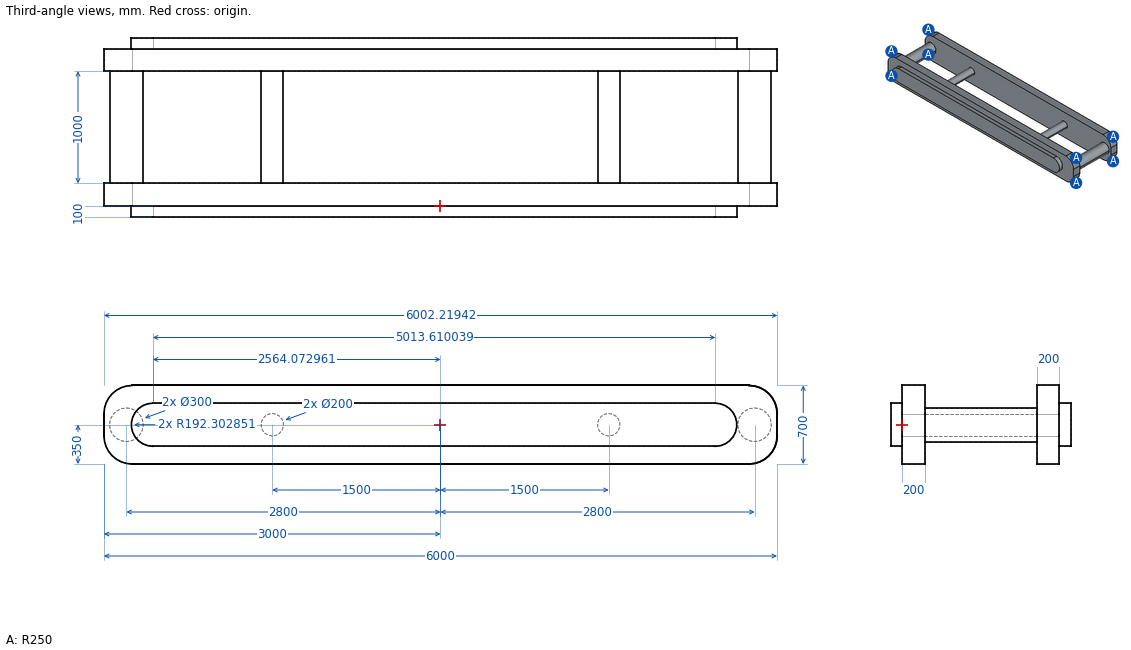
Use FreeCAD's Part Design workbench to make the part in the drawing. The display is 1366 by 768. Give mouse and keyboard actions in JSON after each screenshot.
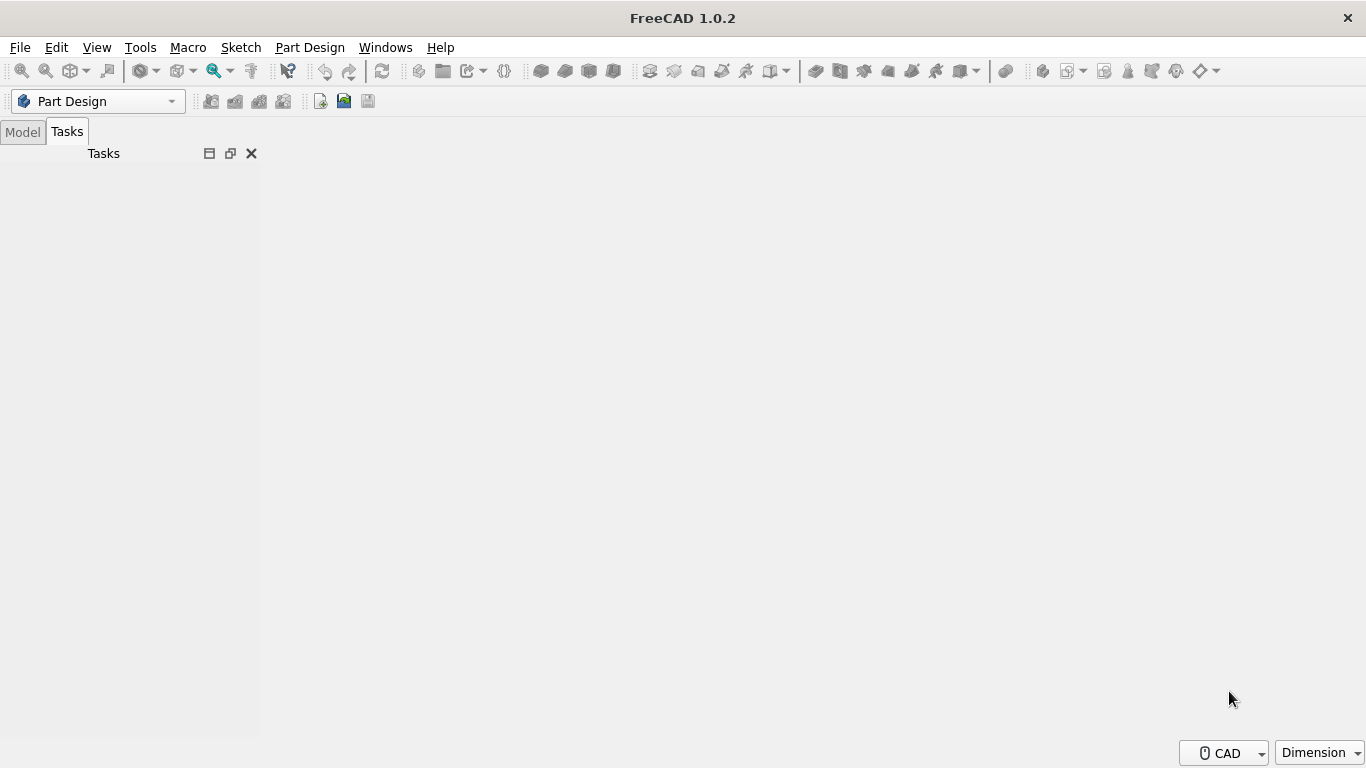
{"action": "left_click", "coordinate": [320, 102]}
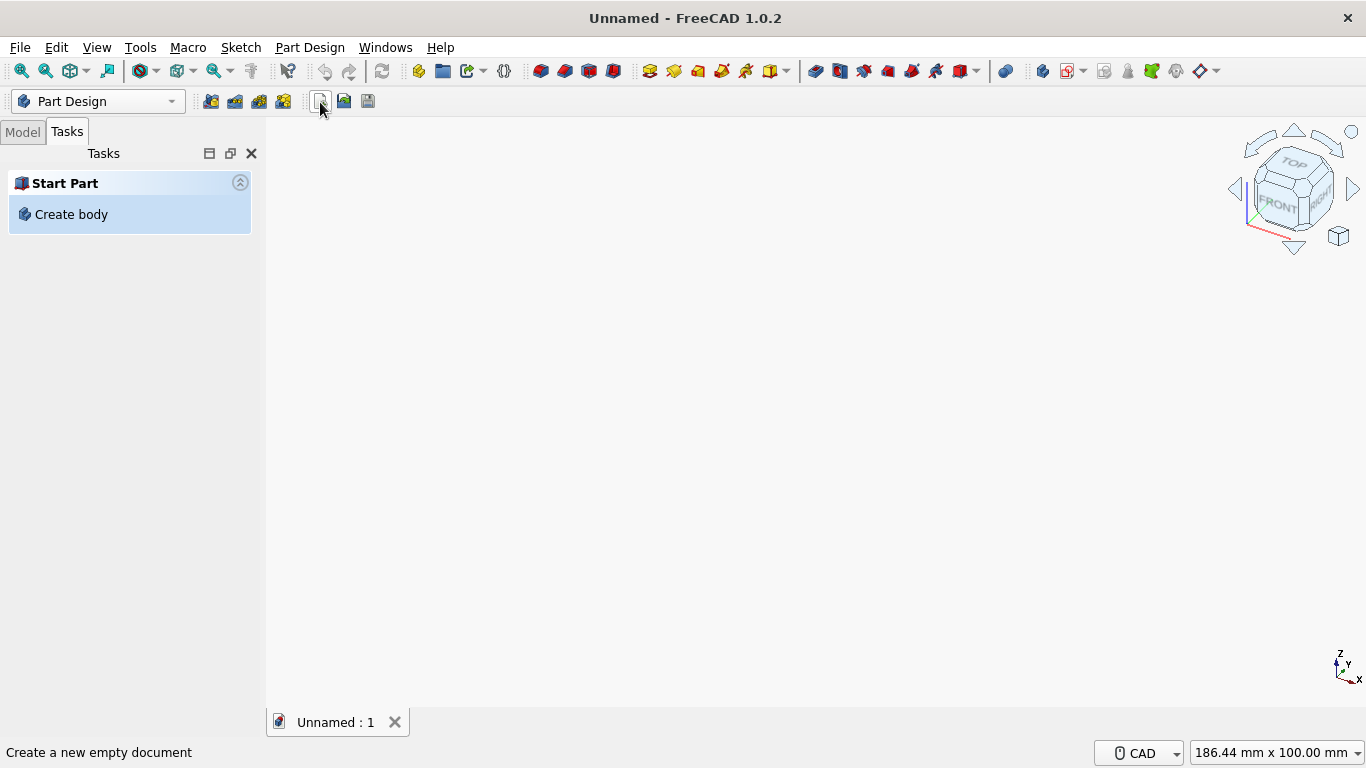
{"action": "left_click", "coordinate": [1068, 72]}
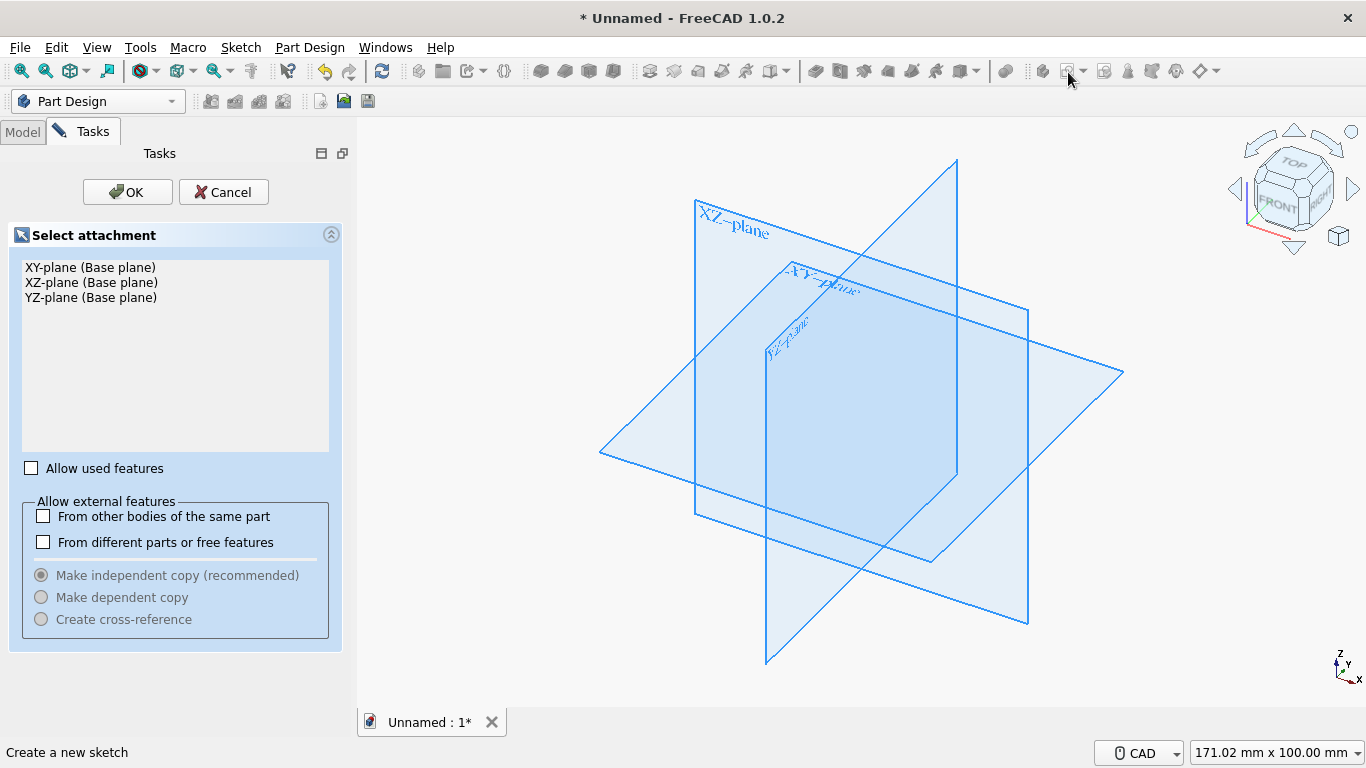
{"action": "left_click", "coordinate": [82, 282]}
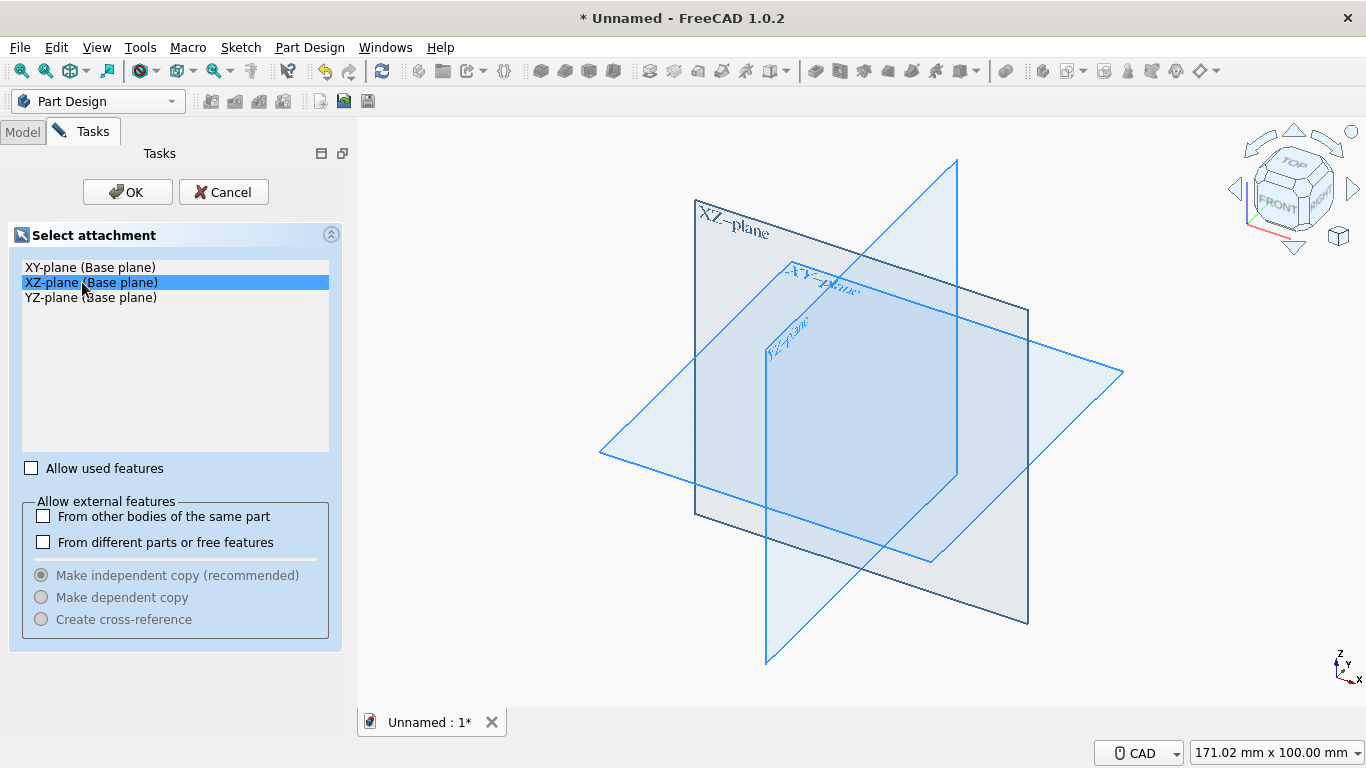
{"action": "left_click", "coordinate": [128, 192]}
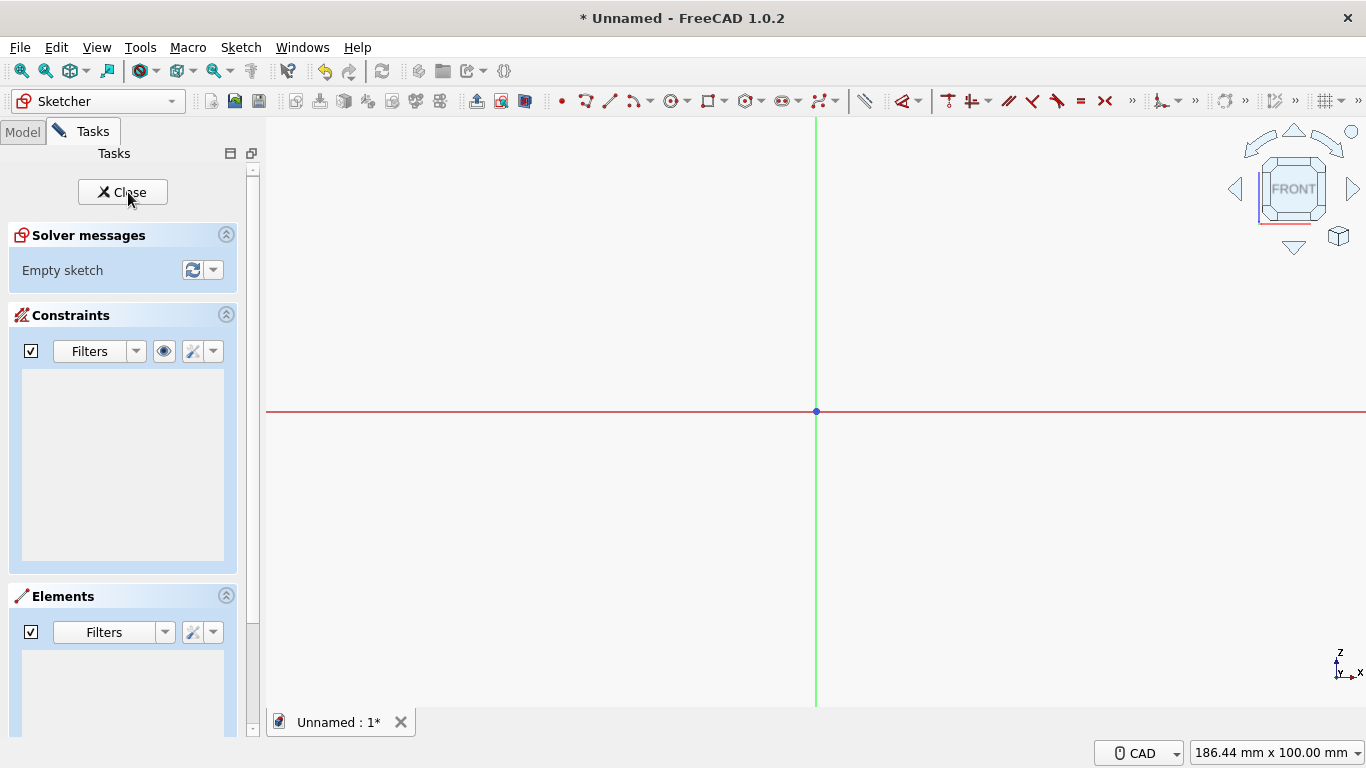
{"action": "scroll", "coordinate": [748, 412], "scroll_direction": "down", "scroll_amount": 15}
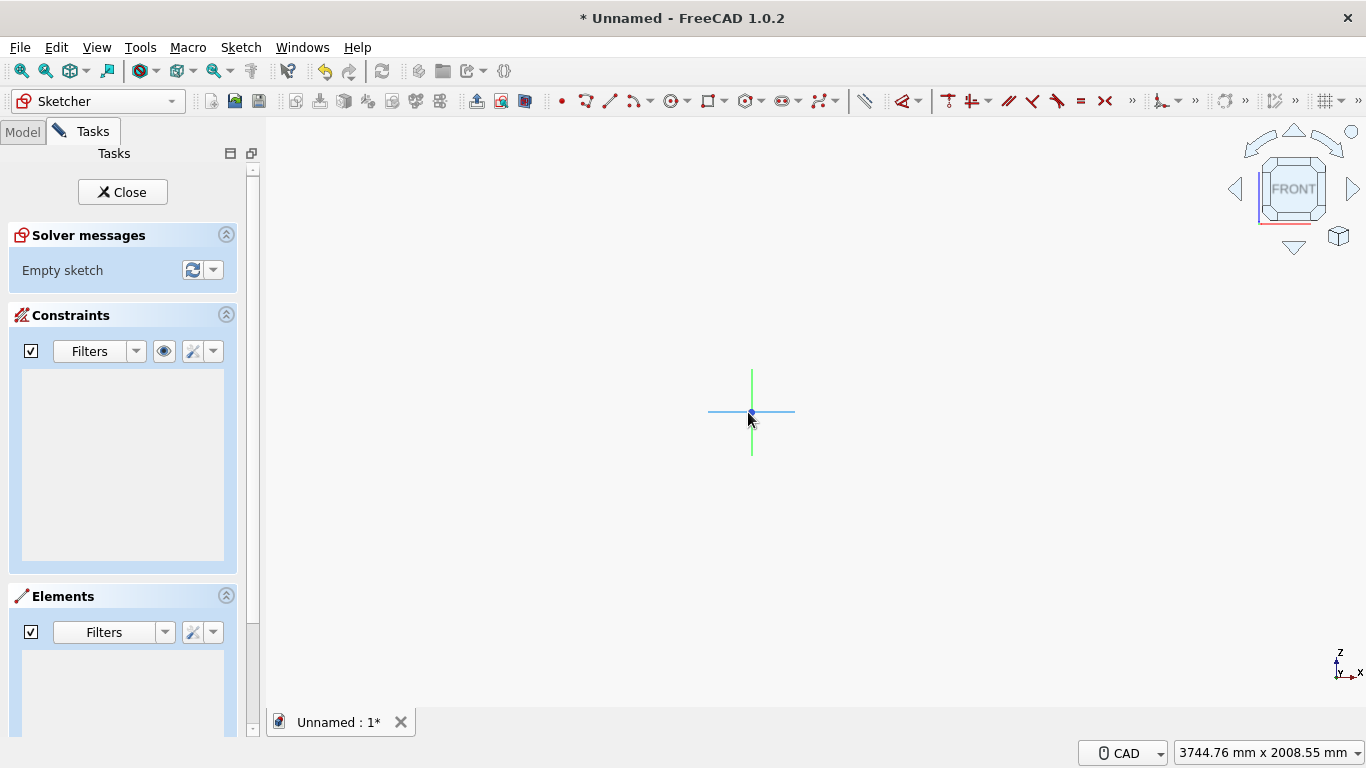
{"action": "scroll", "coordinate": [745, 412], "scroll_direction": "down", "scroll_amount": 5}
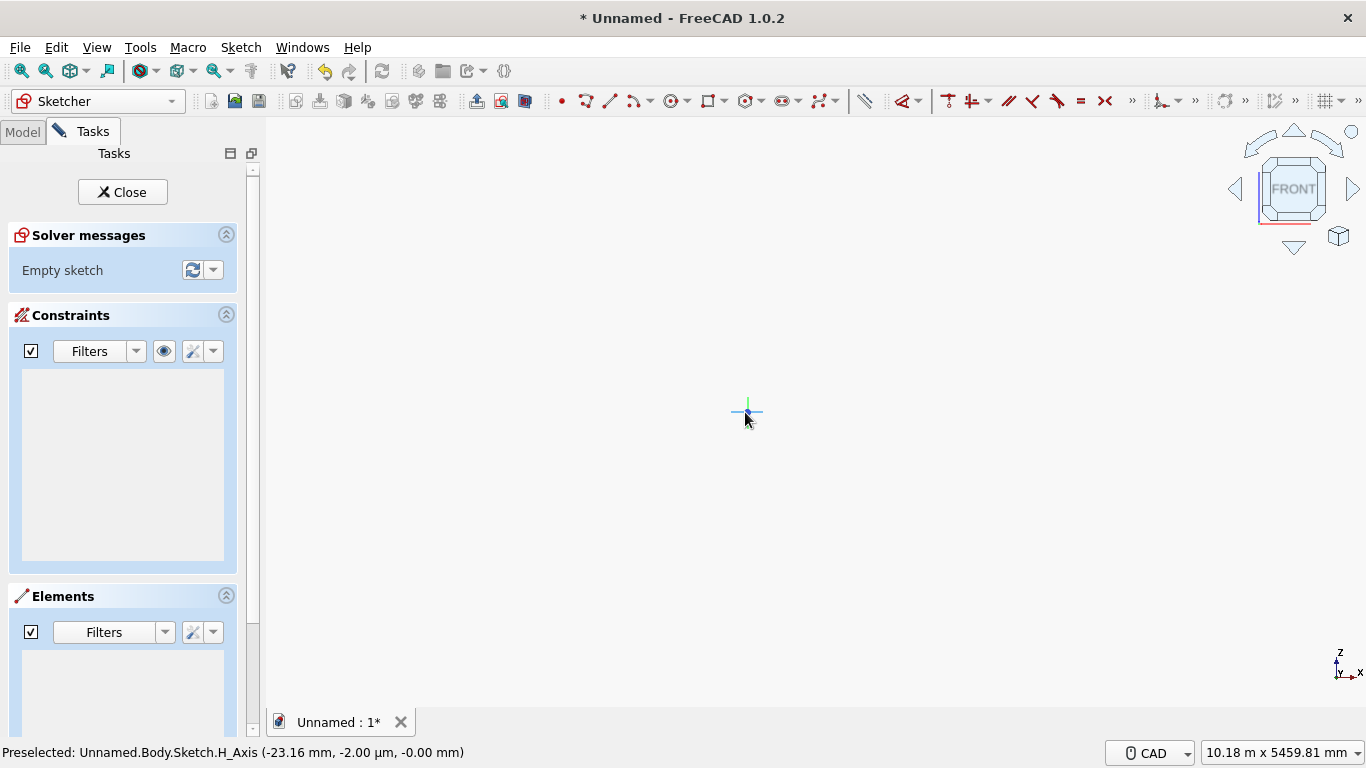
{"action": "key", "text": "g v"}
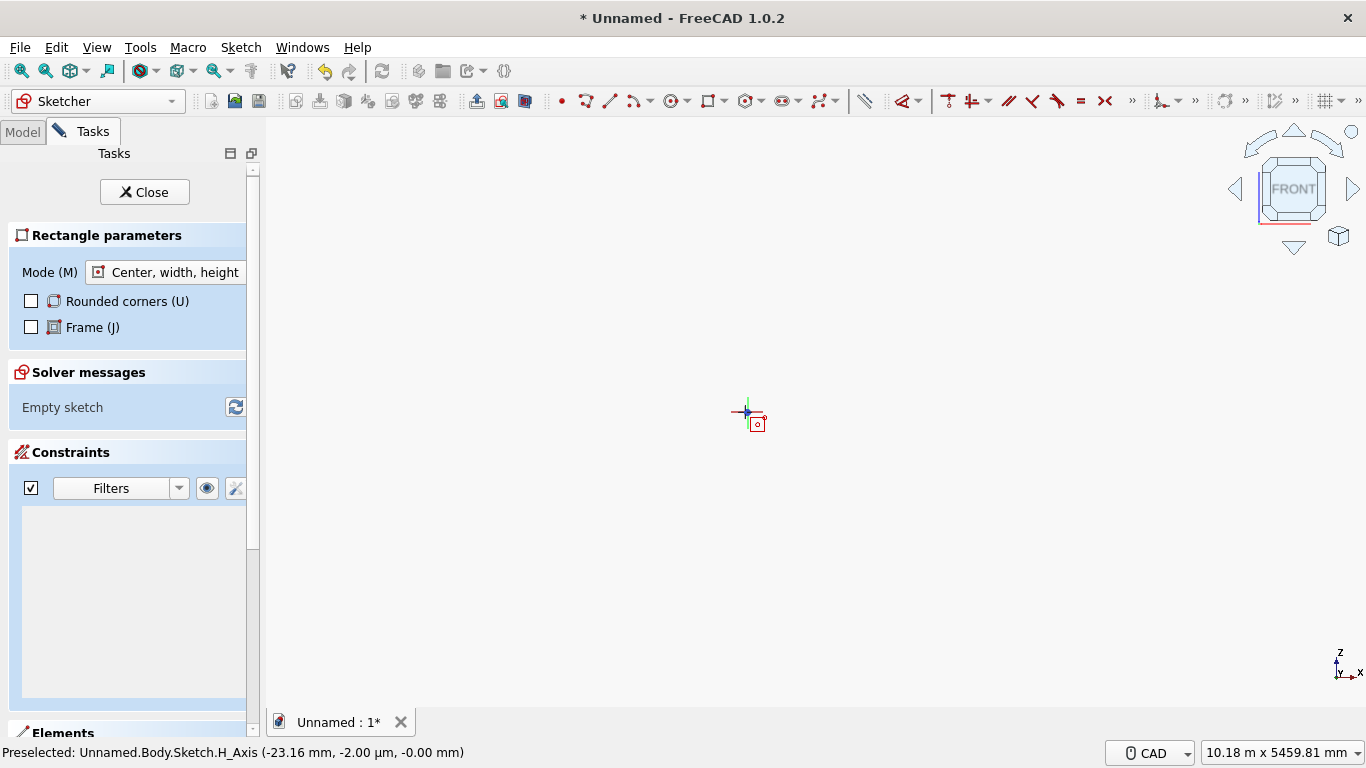
{"action": "left_click", "coordinate": [748, 412]}
{"action": "left_click", "coordinate": [1072, 375]}
{"action": "key", "text": "Escape"}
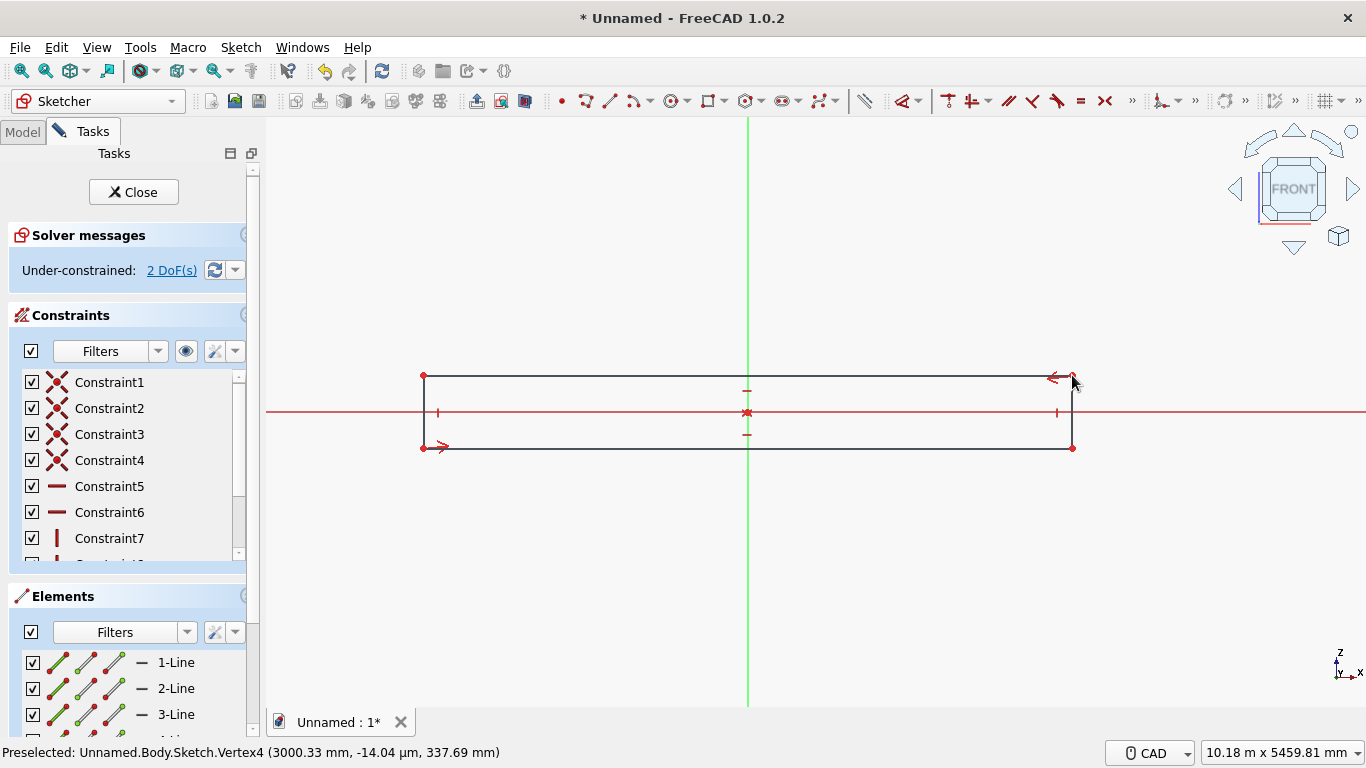
{"action": "left_click", "coordinate": [1072, 427]}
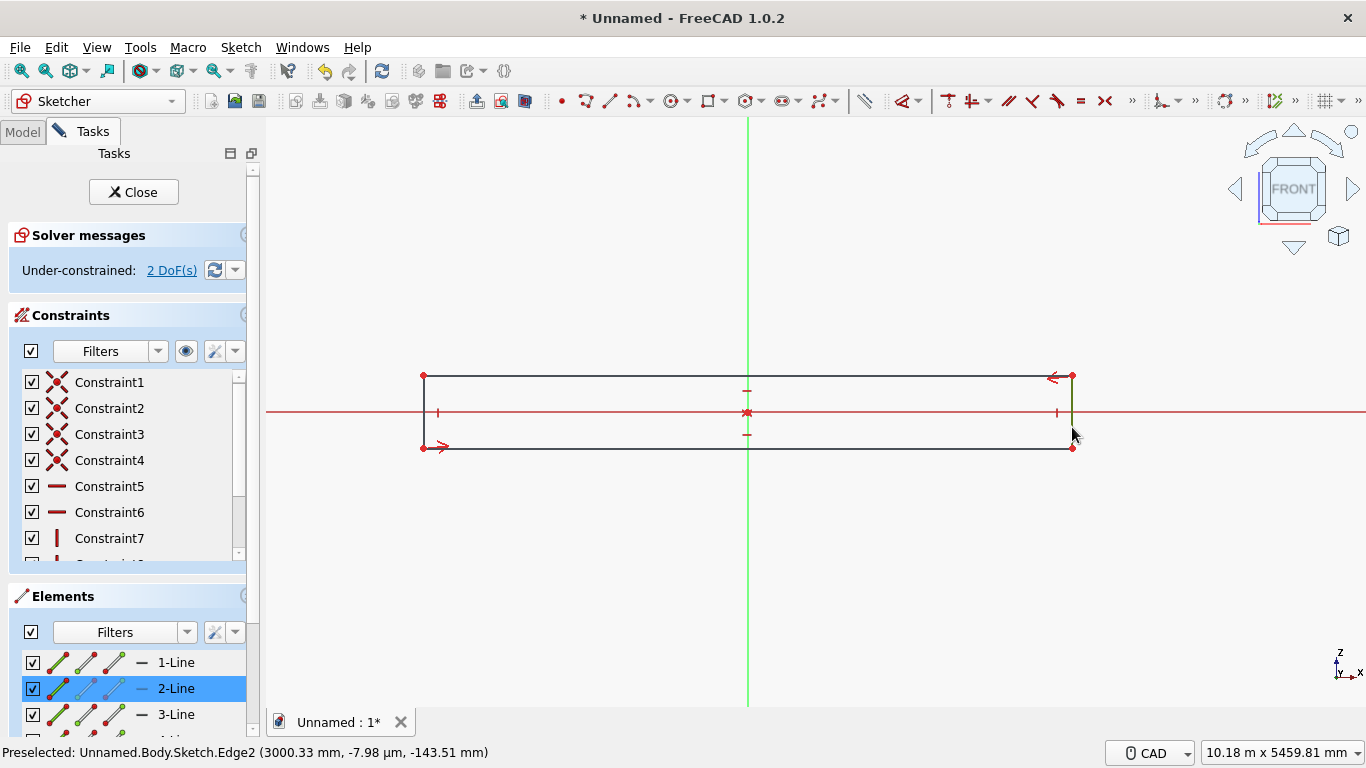
{"action": "key", "text": "i"}